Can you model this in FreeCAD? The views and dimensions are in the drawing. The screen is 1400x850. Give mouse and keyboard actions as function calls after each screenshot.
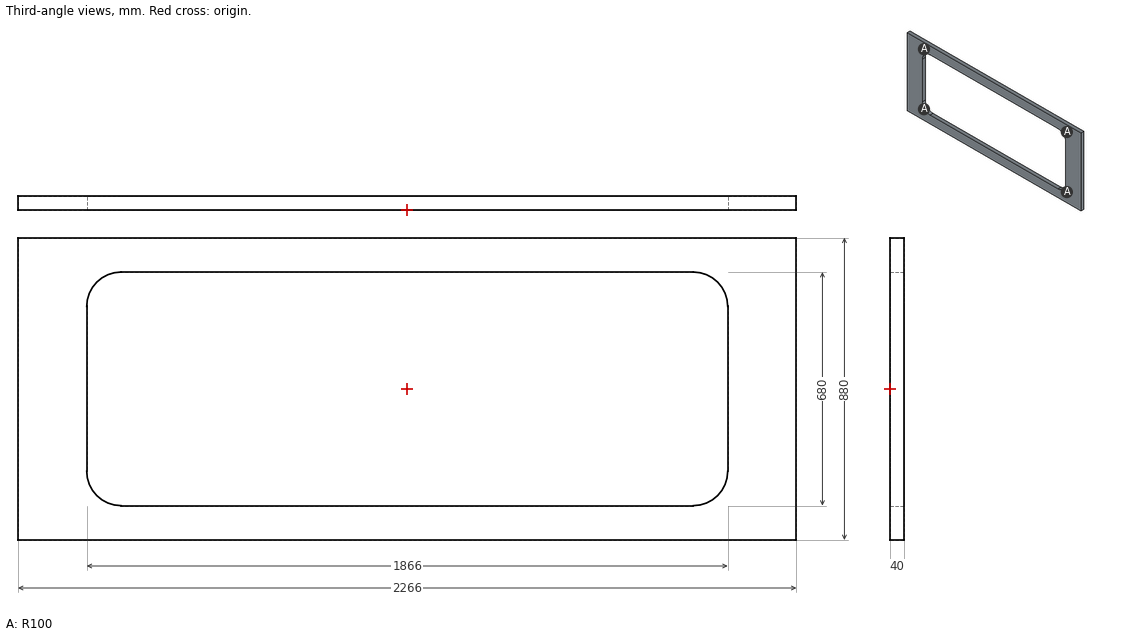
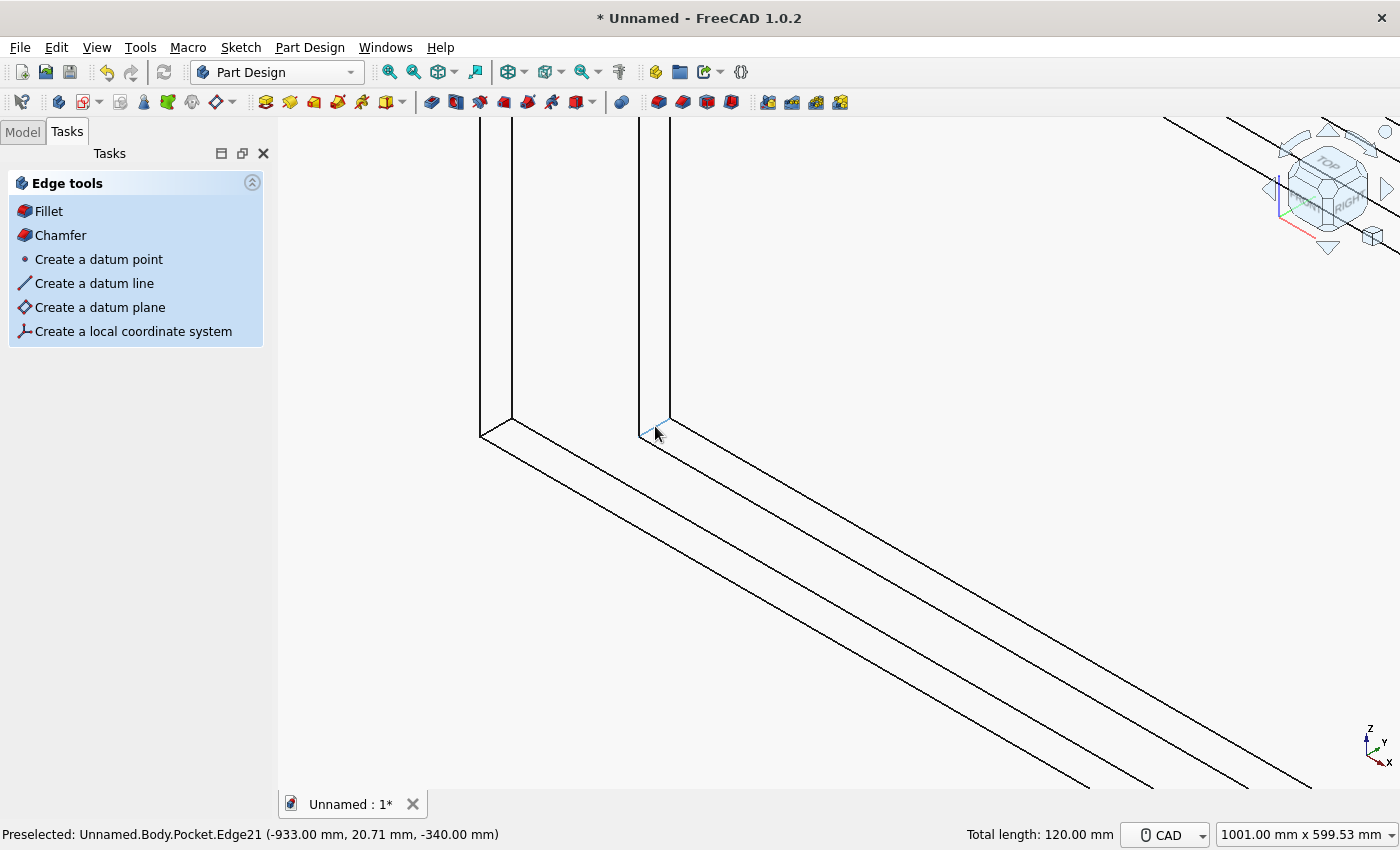
click(390, 72)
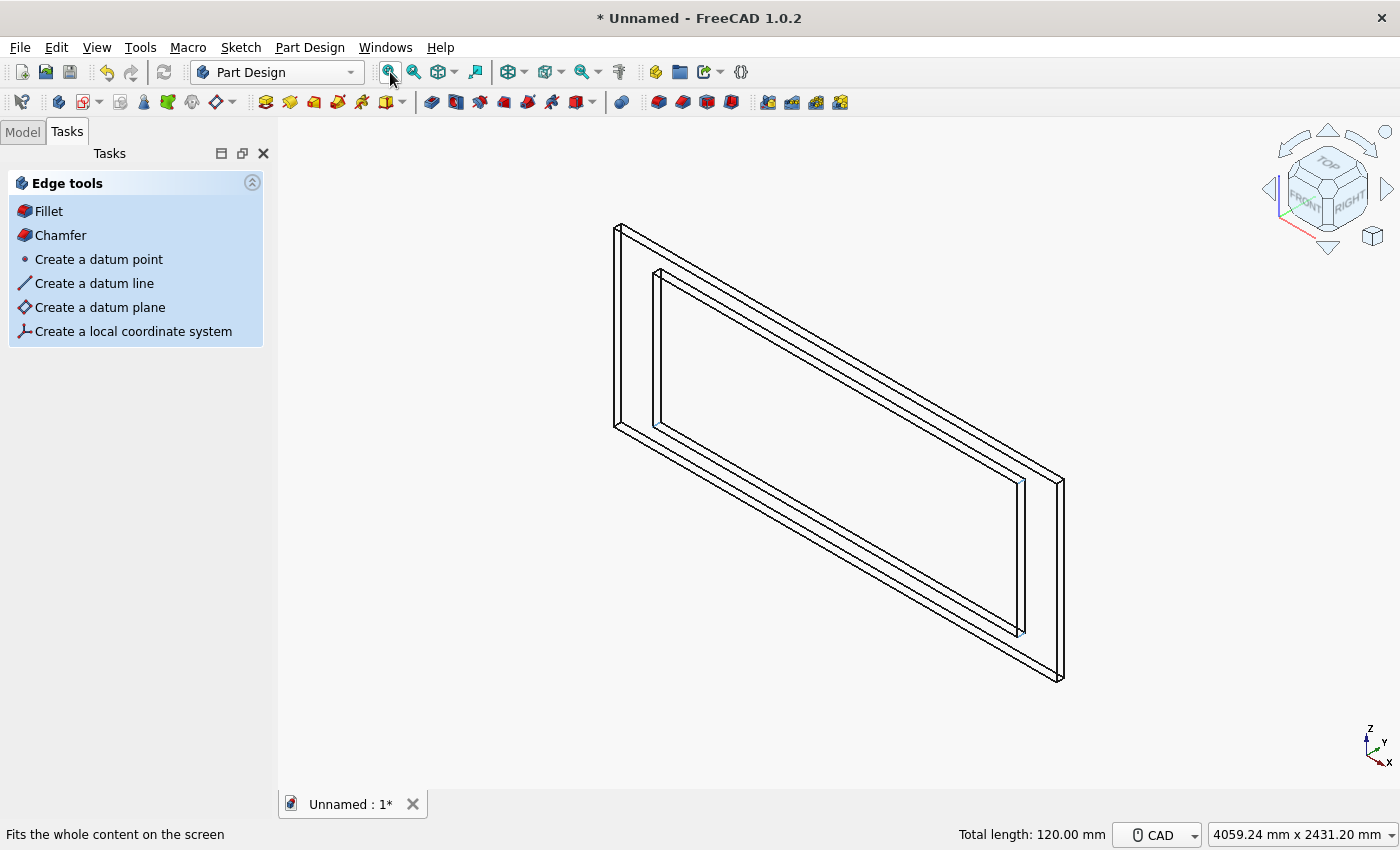
key(2)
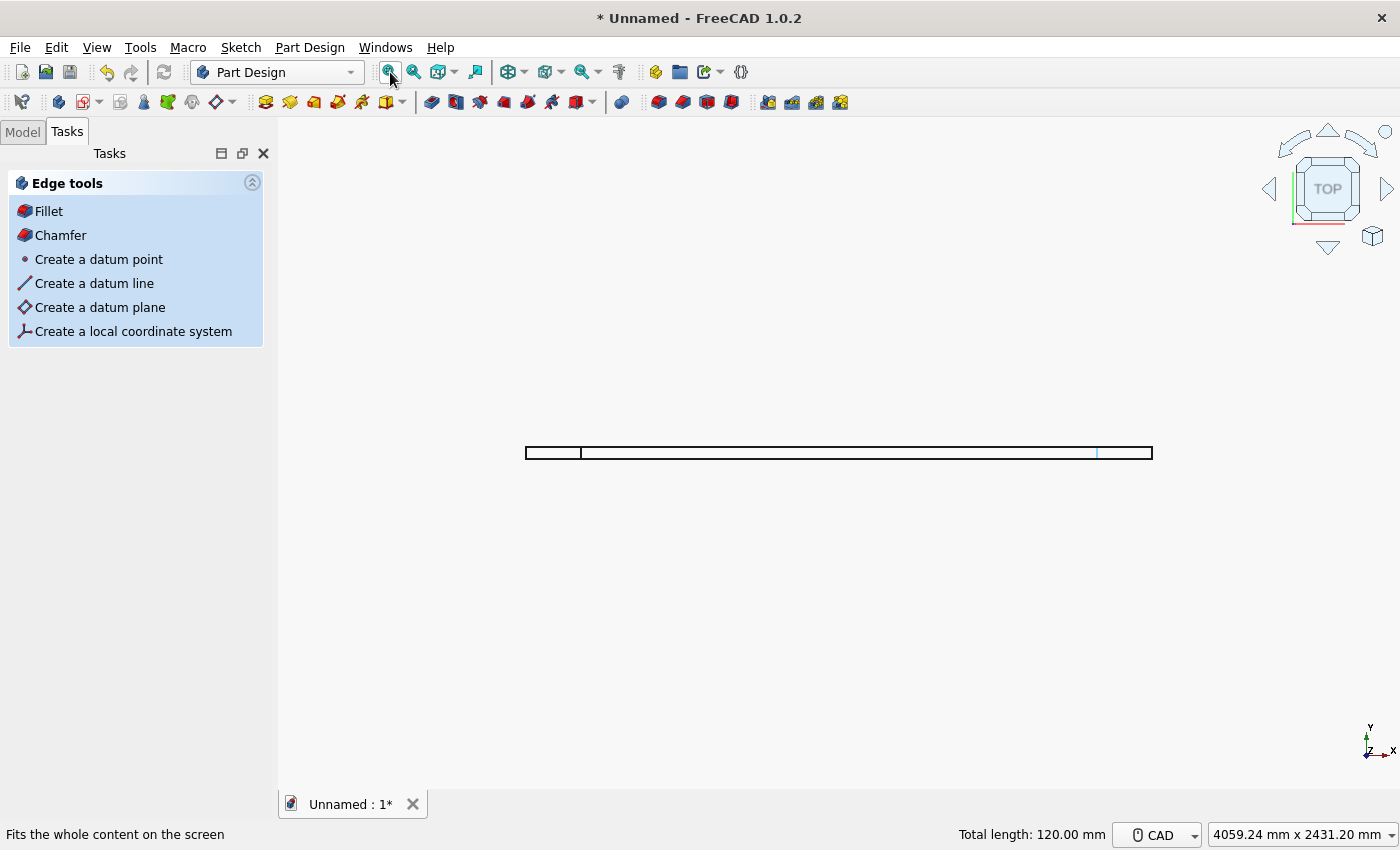
scroll(581, 452, up, 7)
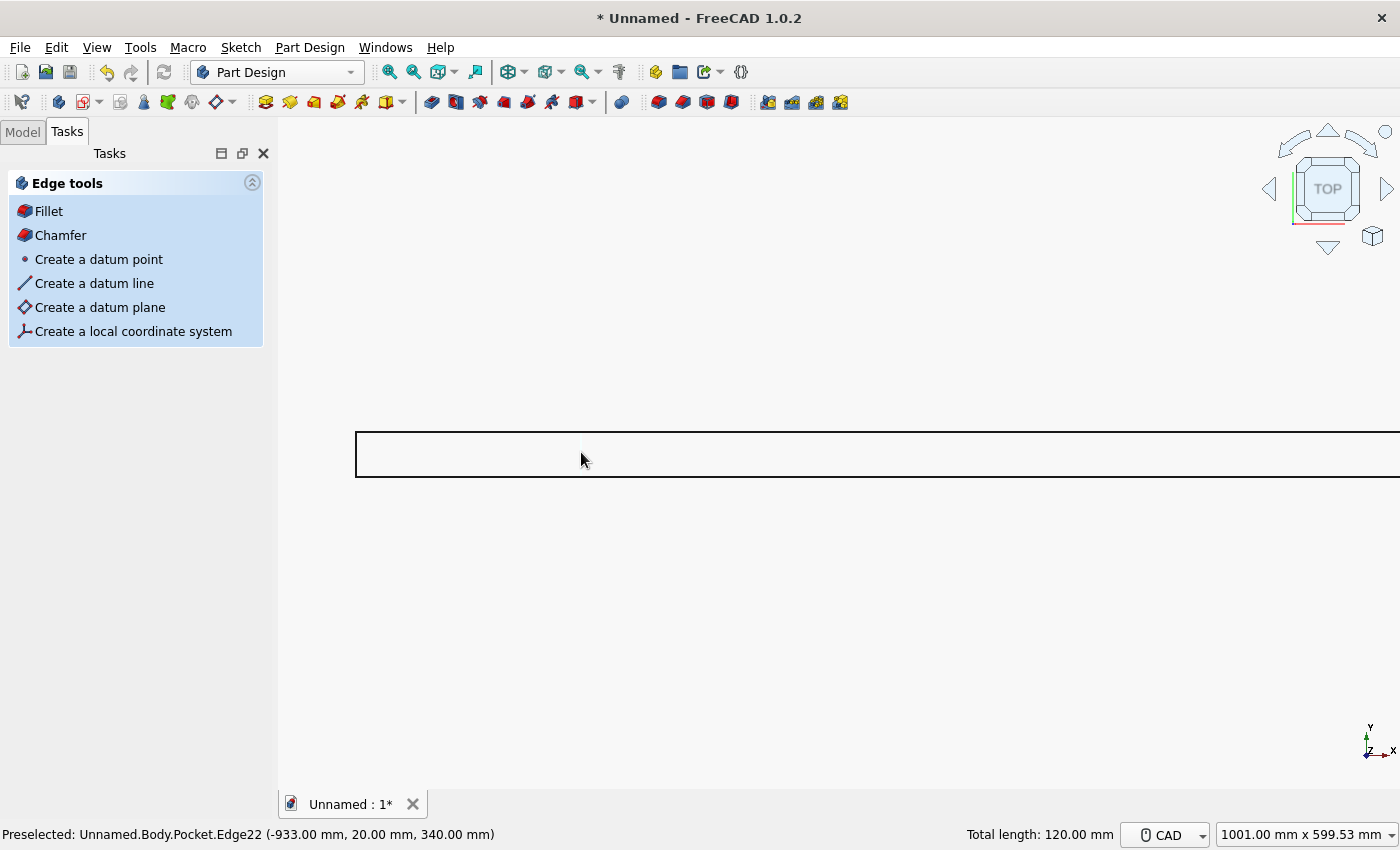
click(581, 454, ctrl)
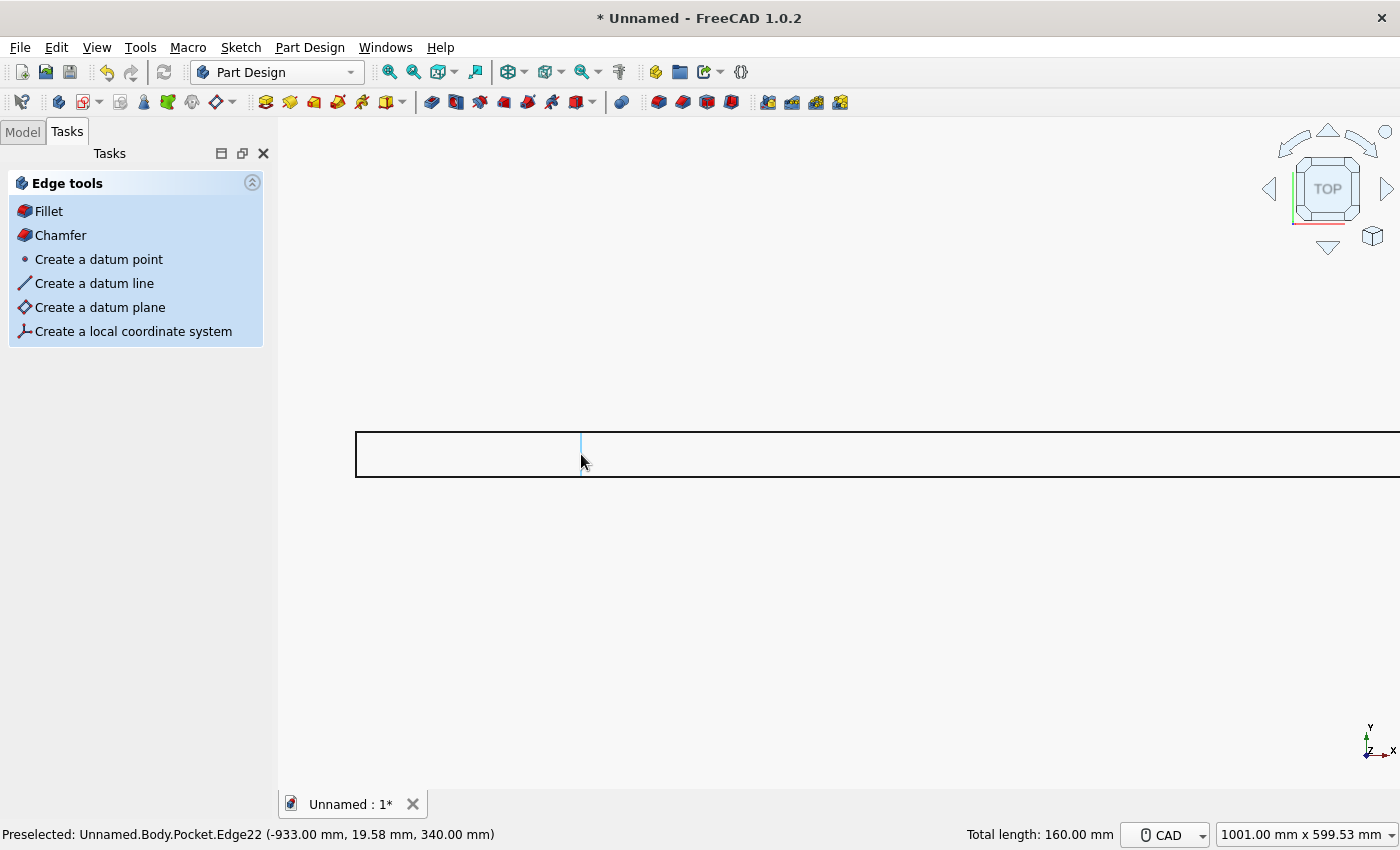
key(v)
key(1)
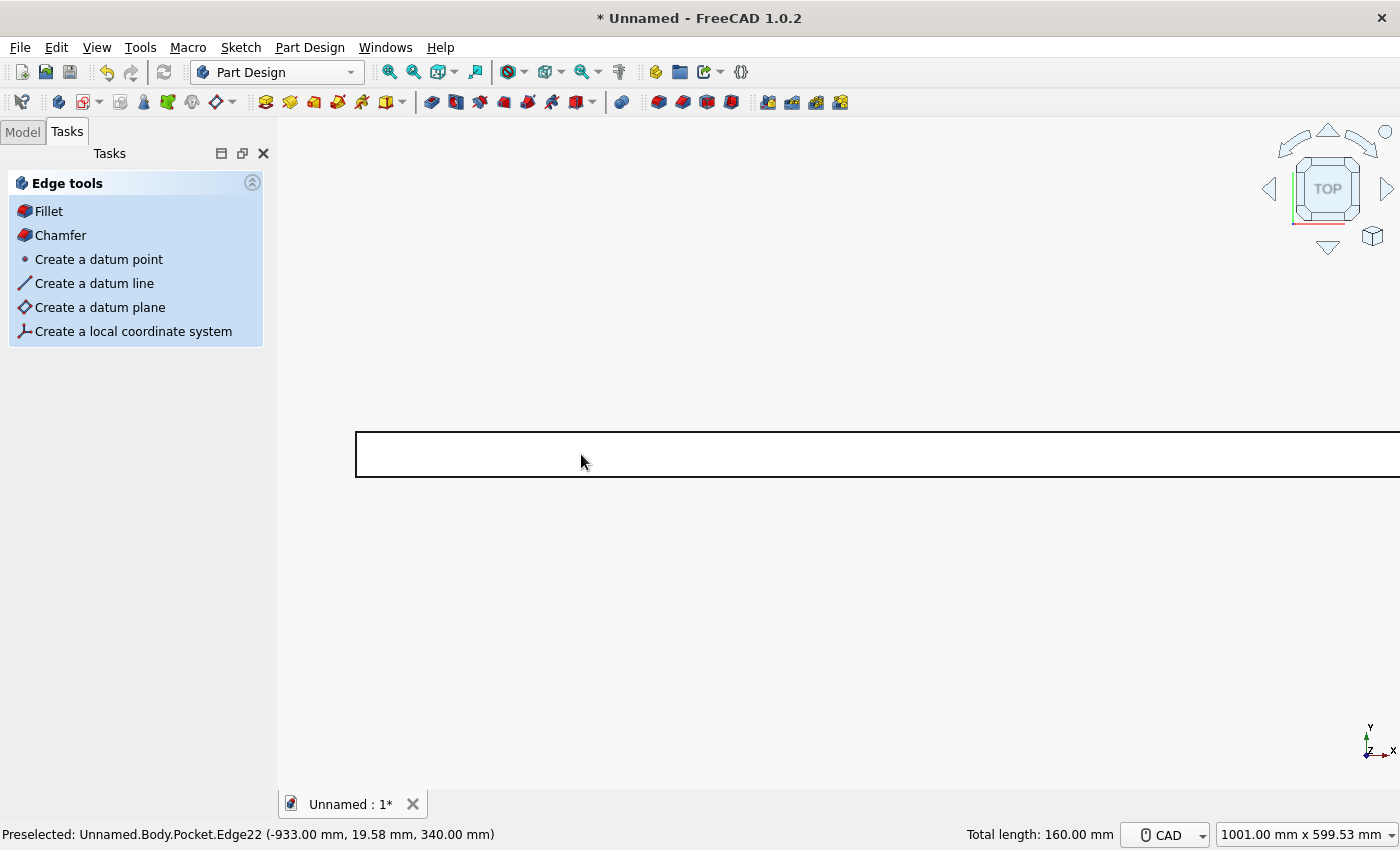
click(660, 102)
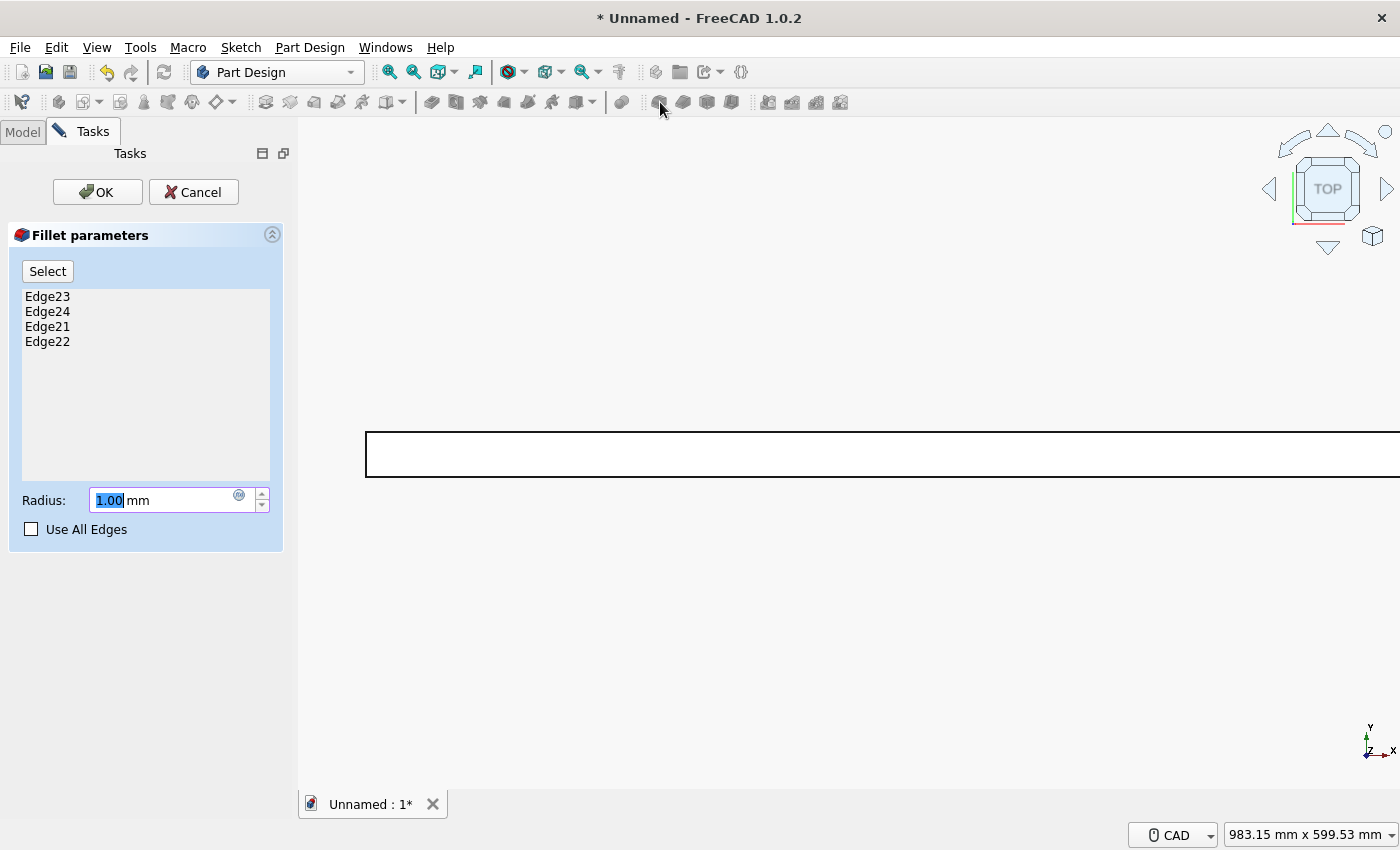
text(100)
key(Tab)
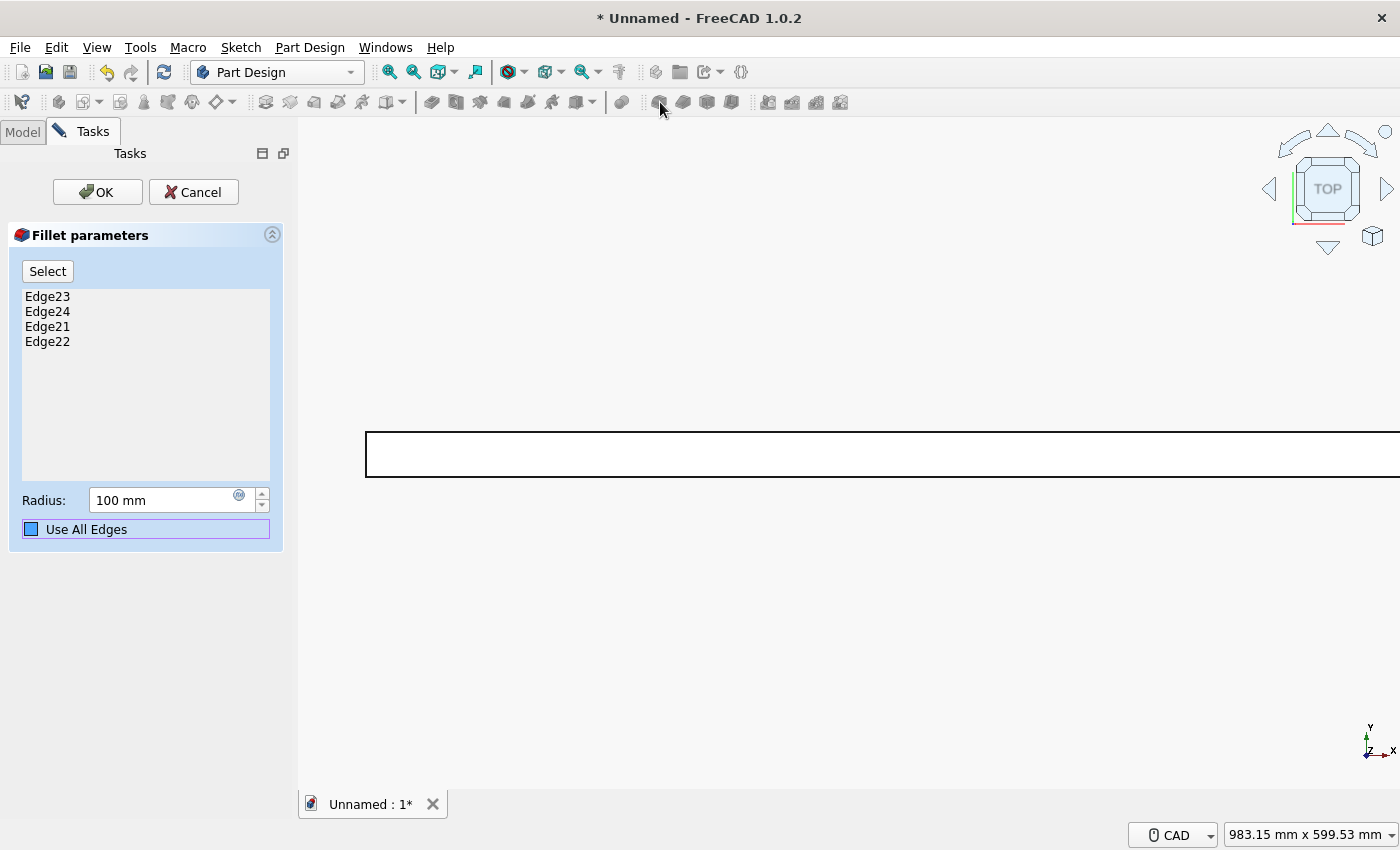
click(98, 192)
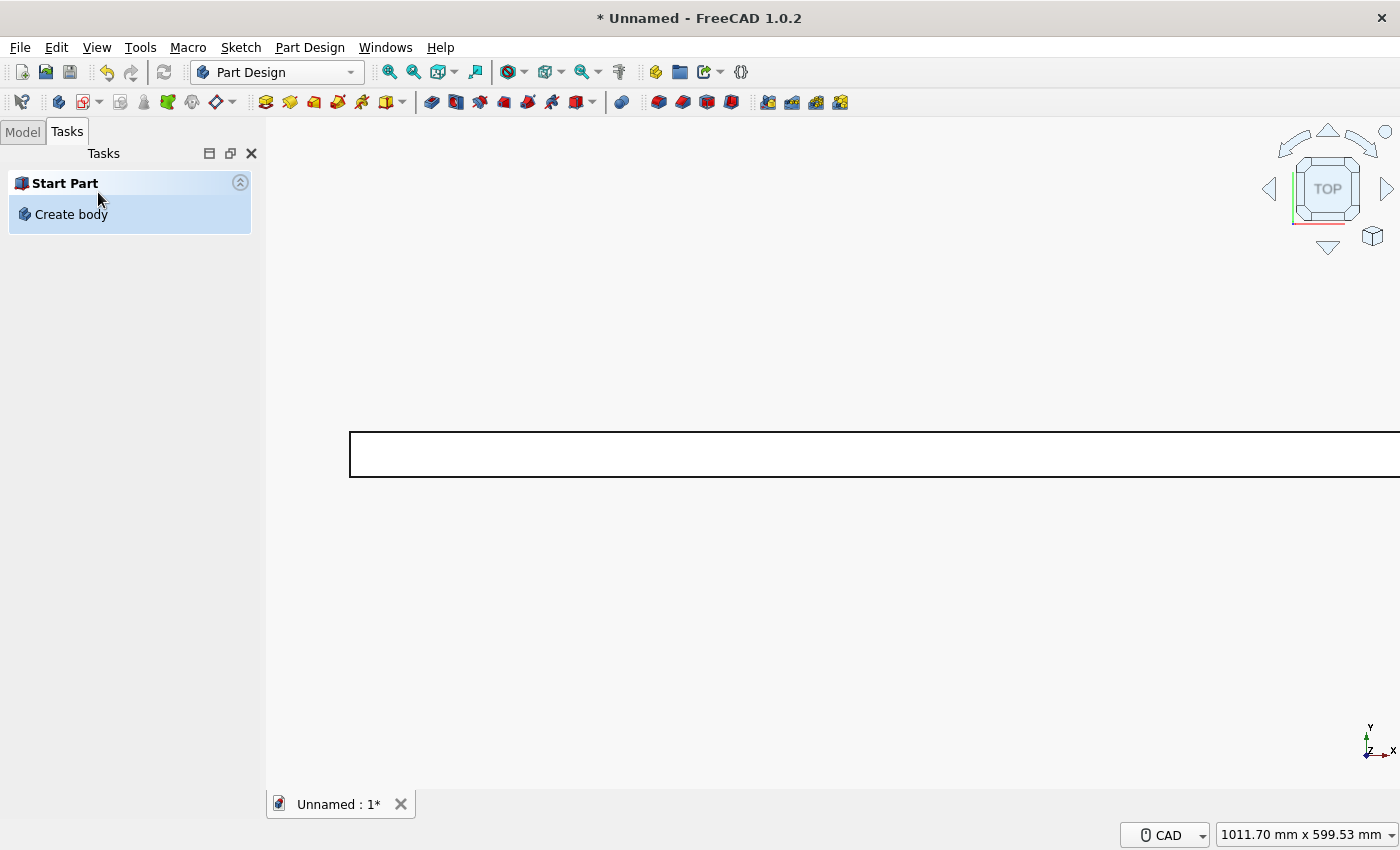
key(0)